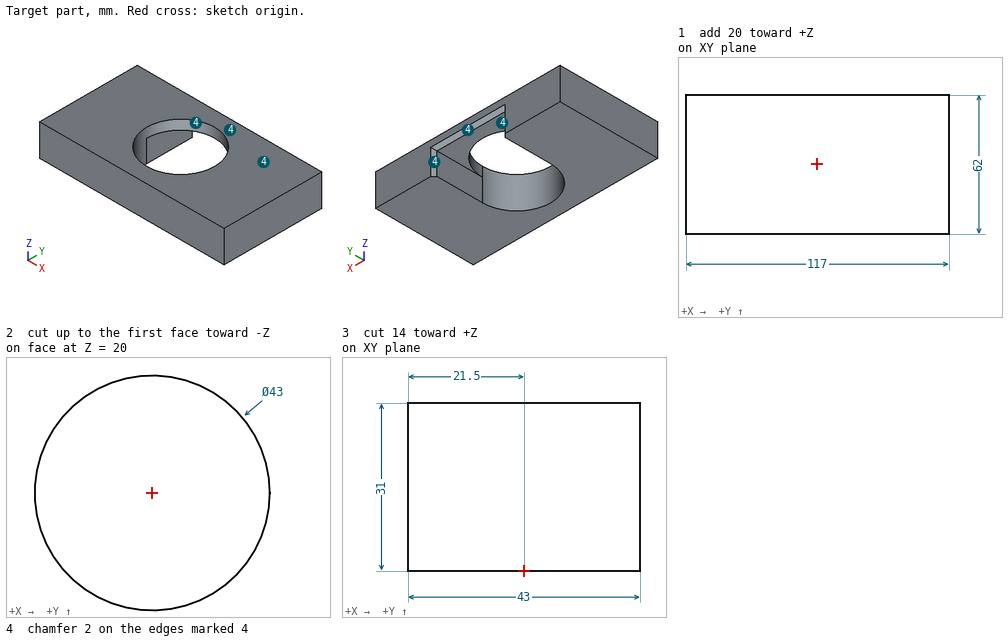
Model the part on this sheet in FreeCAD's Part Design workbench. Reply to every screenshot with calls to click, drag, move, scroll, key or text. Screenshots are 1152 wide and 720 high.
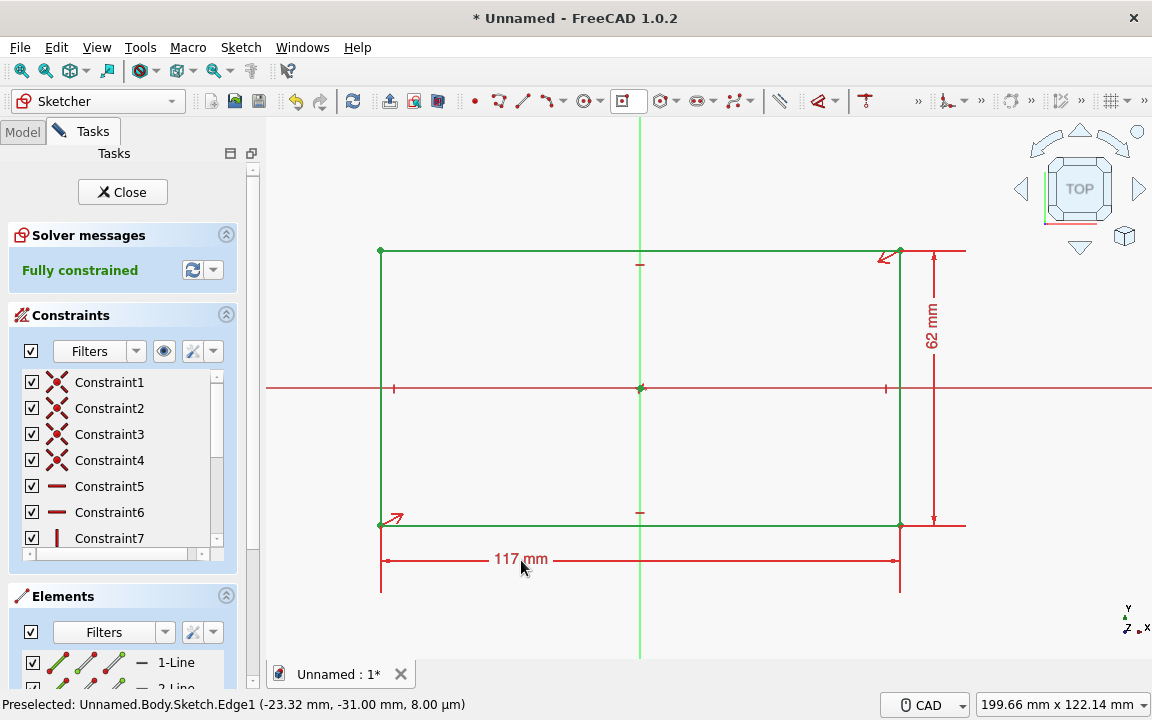
click(123, 192)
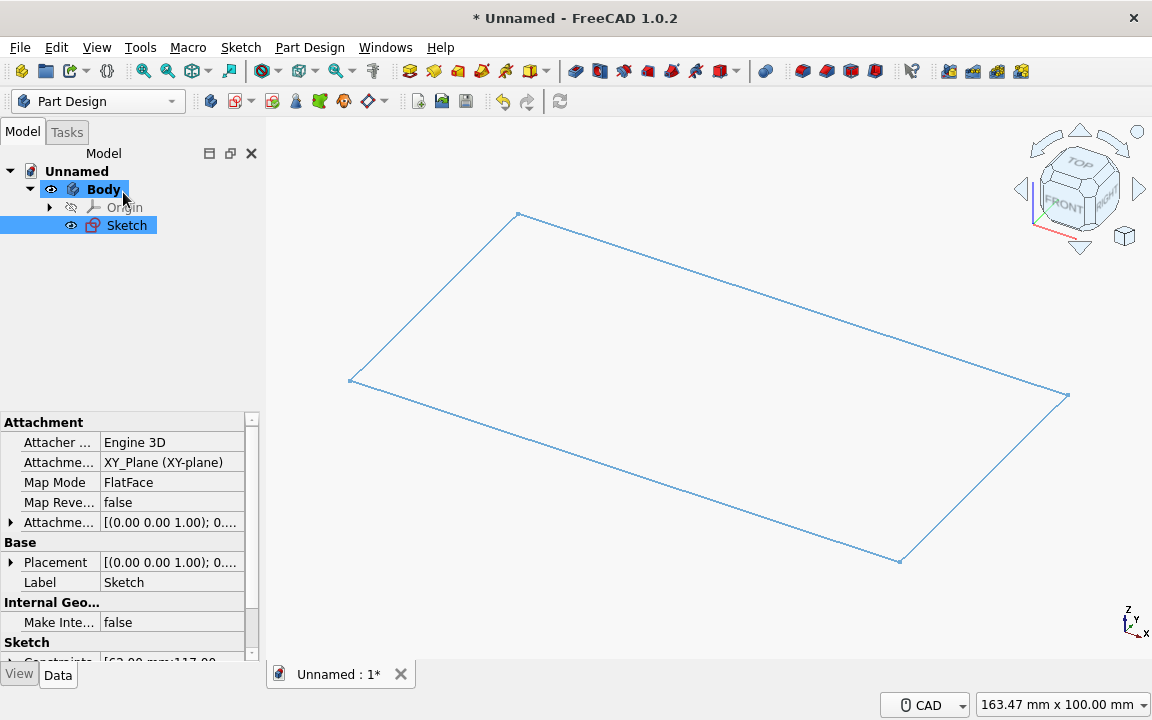
click(410, 72)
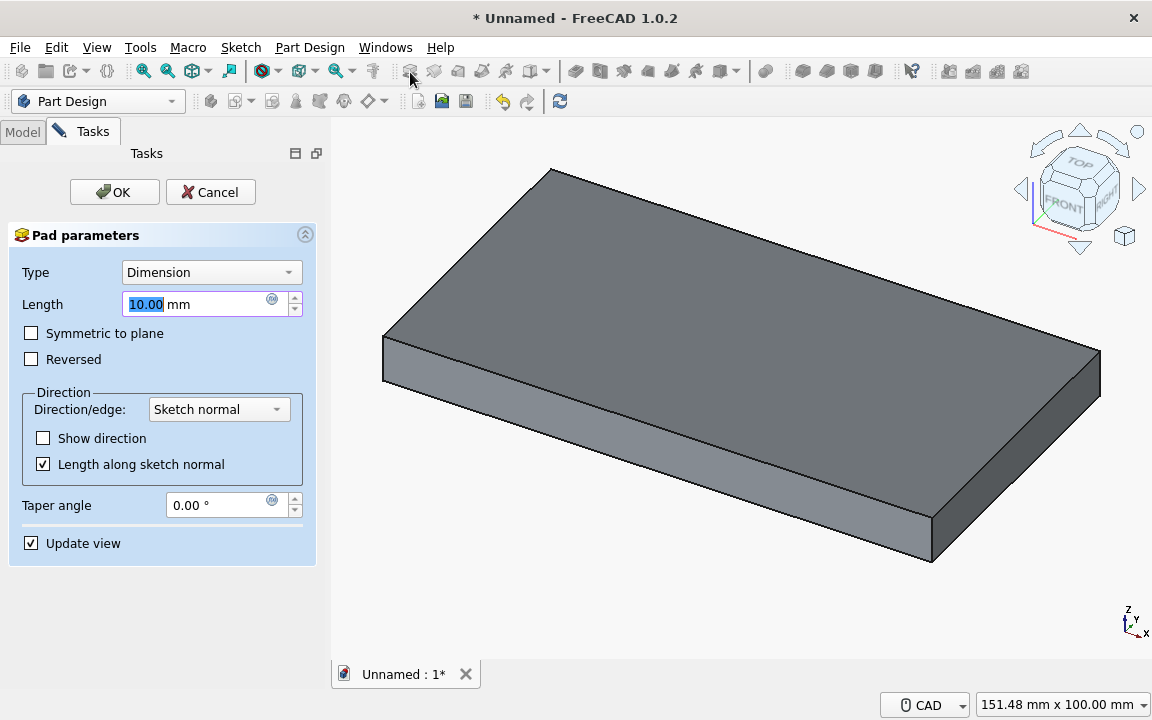
text(20)
key(Tab)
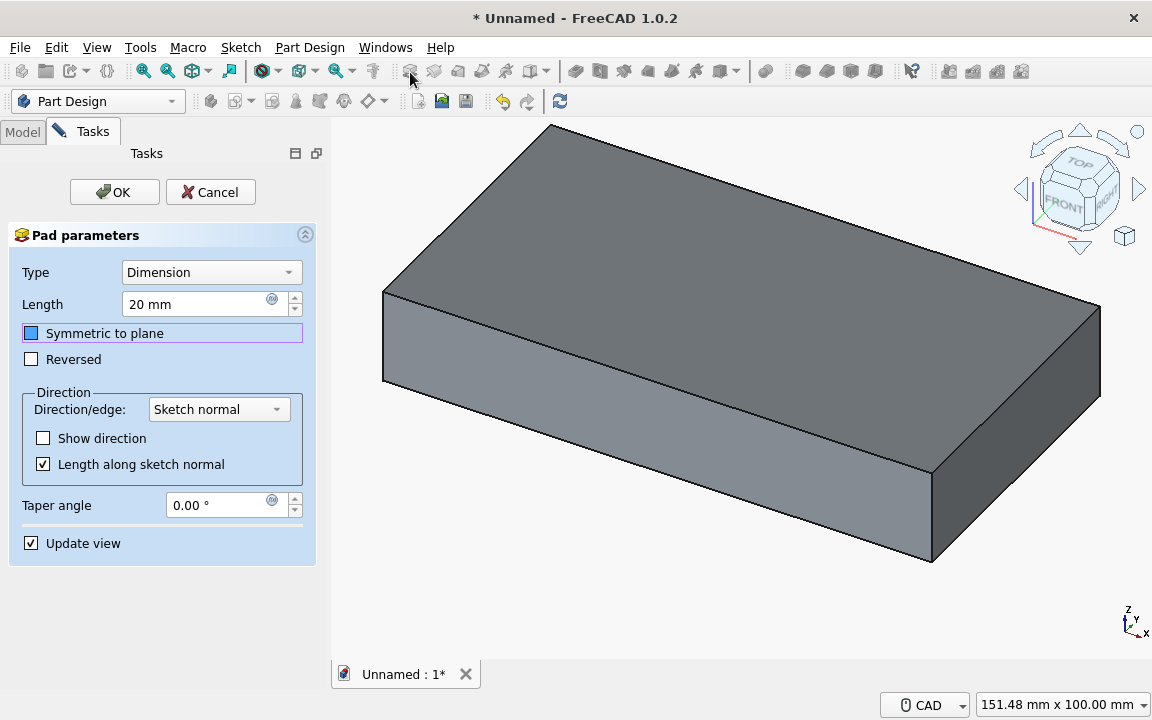
click(115, 192)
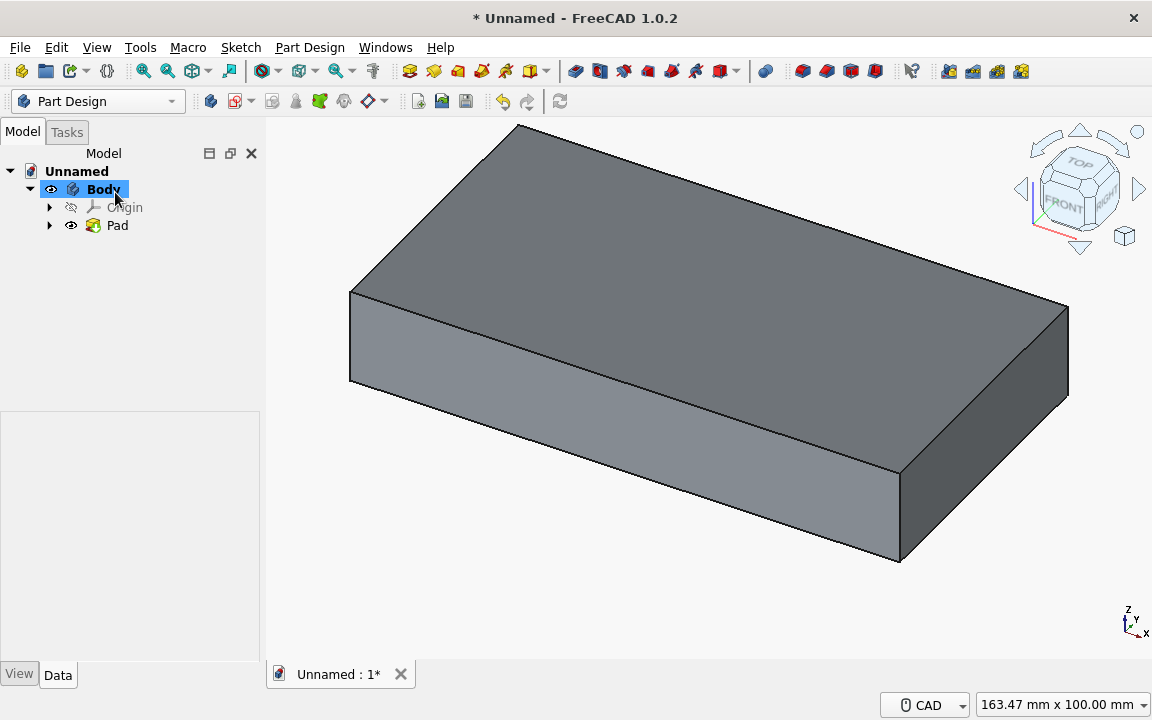
click(787, 324)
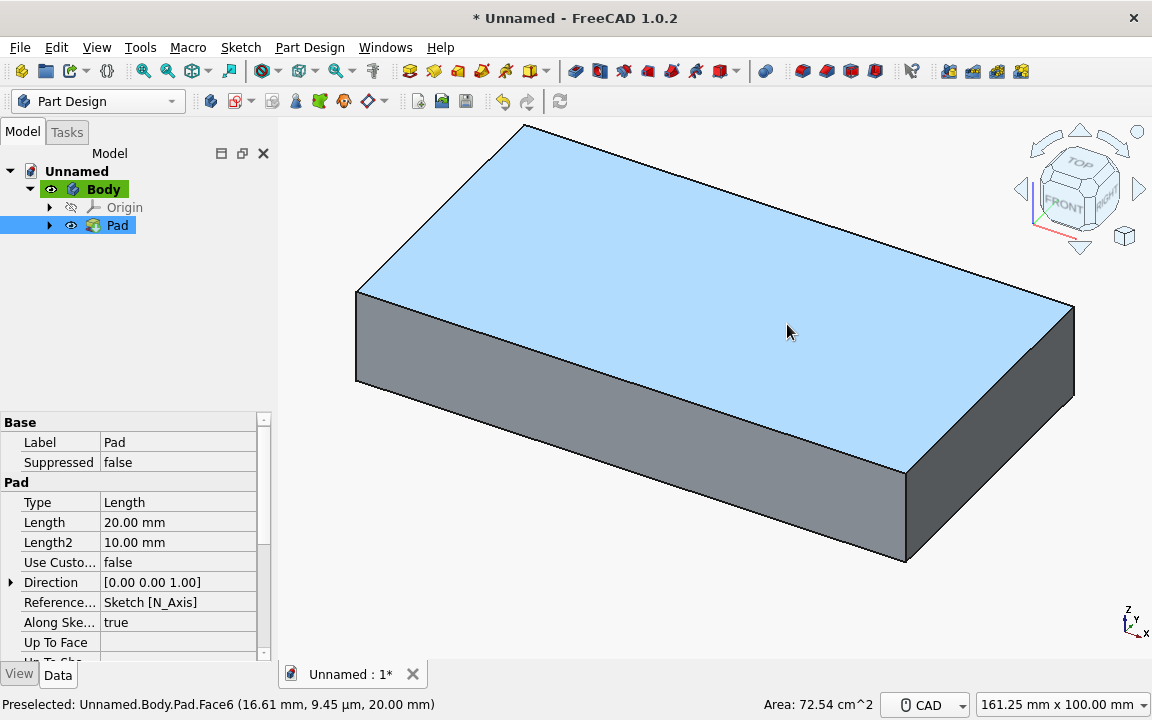
click(236, 102)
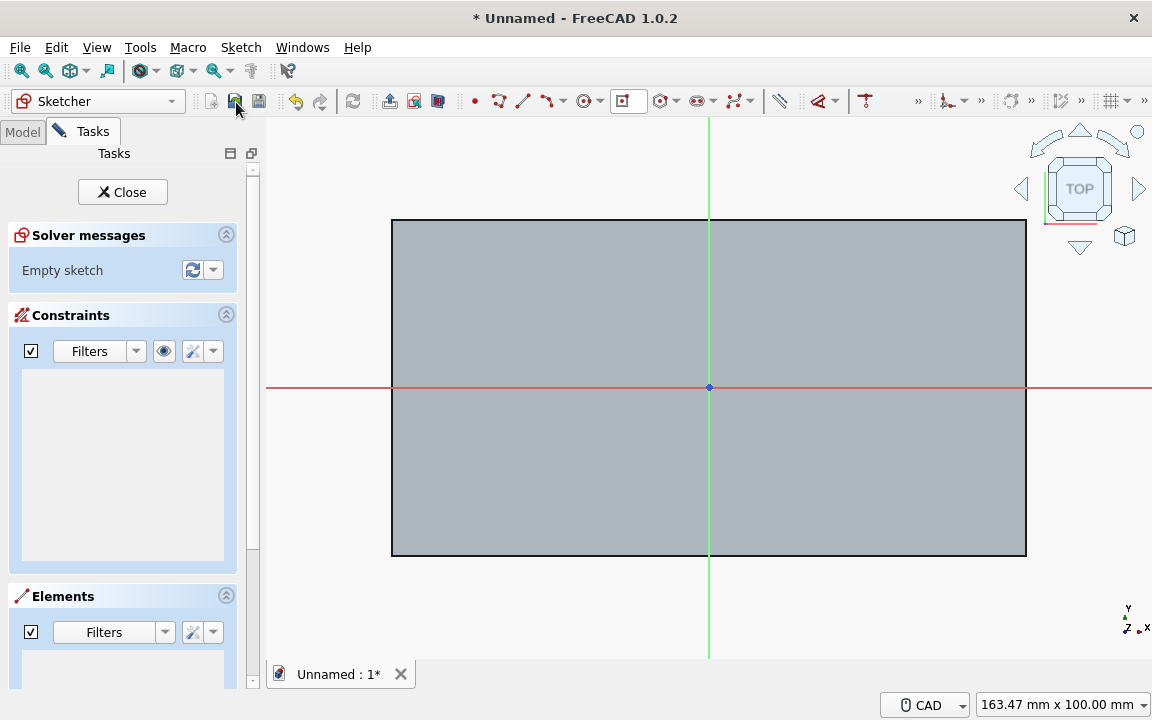
scroll(848, 388, up, 2)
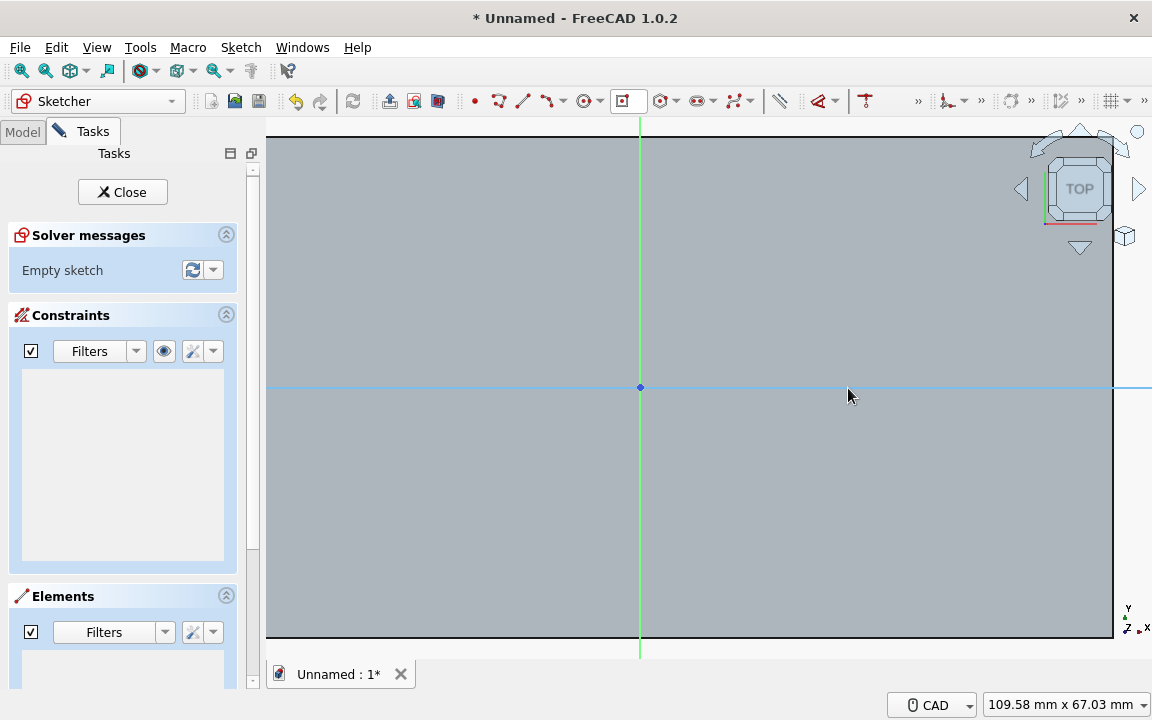
key(g)
key(c)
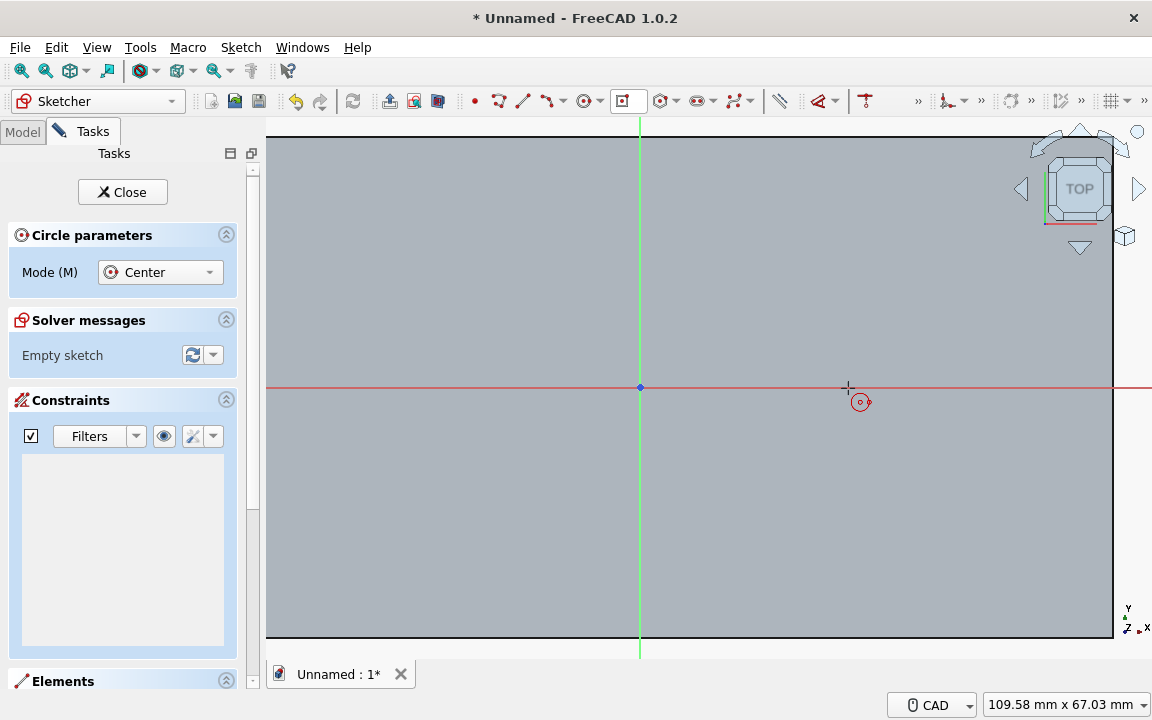
click(640, 388)
click(763, 265)
key(Escape)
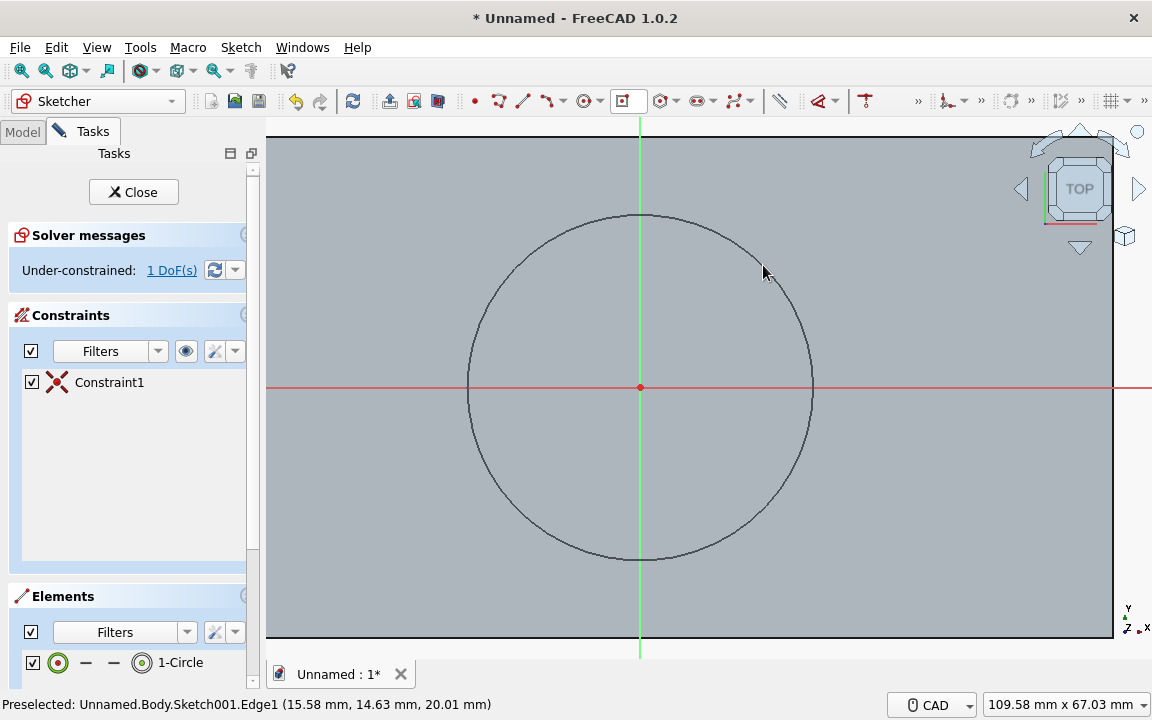
key(d)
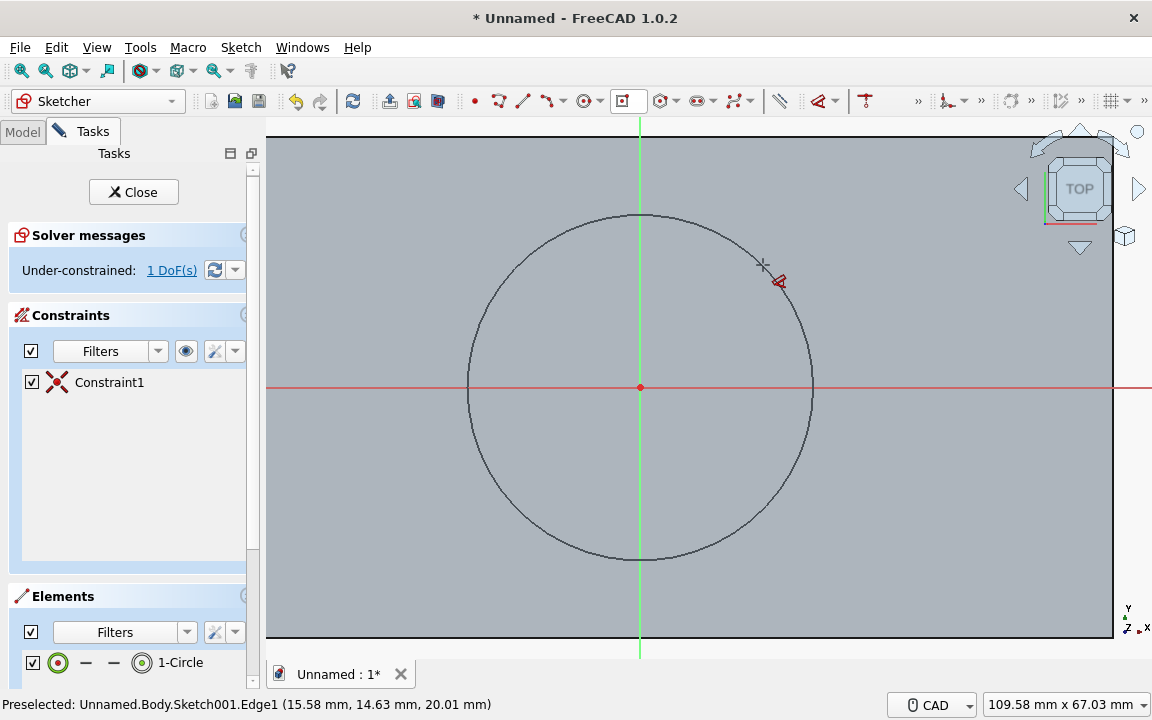
click(762, 265)
click(785, 242)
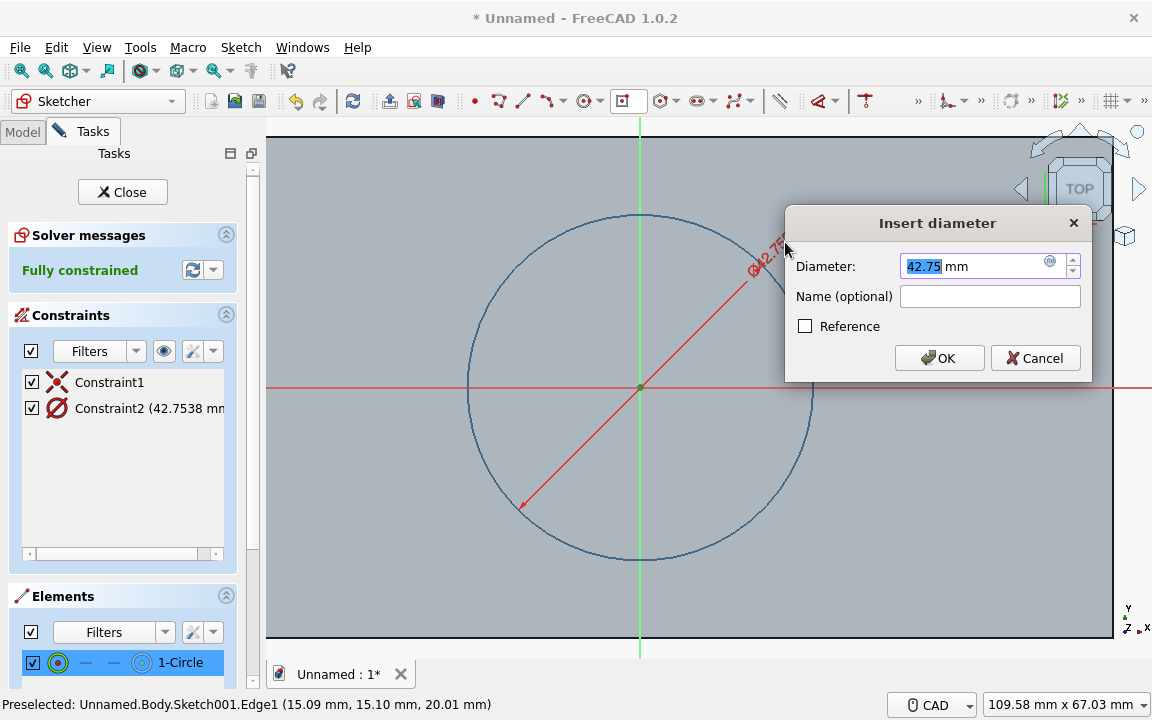
text(43)
key(Return)
key(Escape)